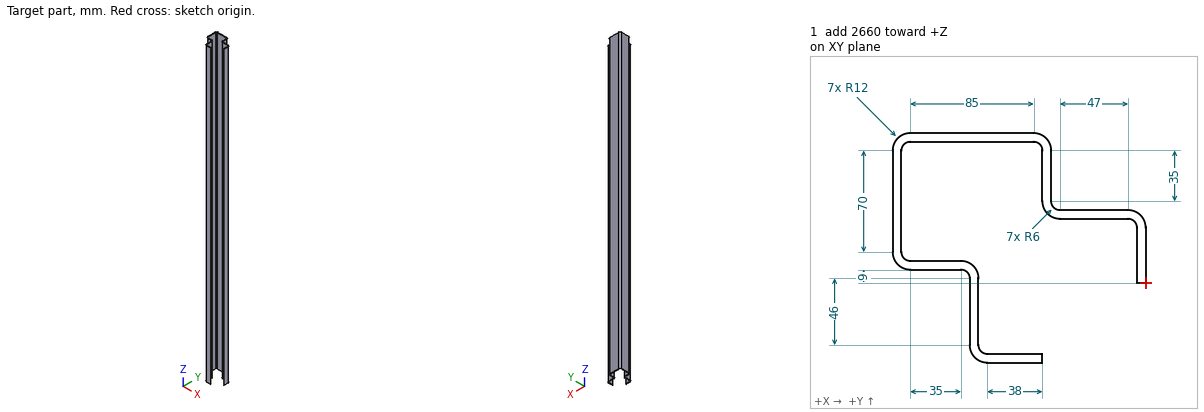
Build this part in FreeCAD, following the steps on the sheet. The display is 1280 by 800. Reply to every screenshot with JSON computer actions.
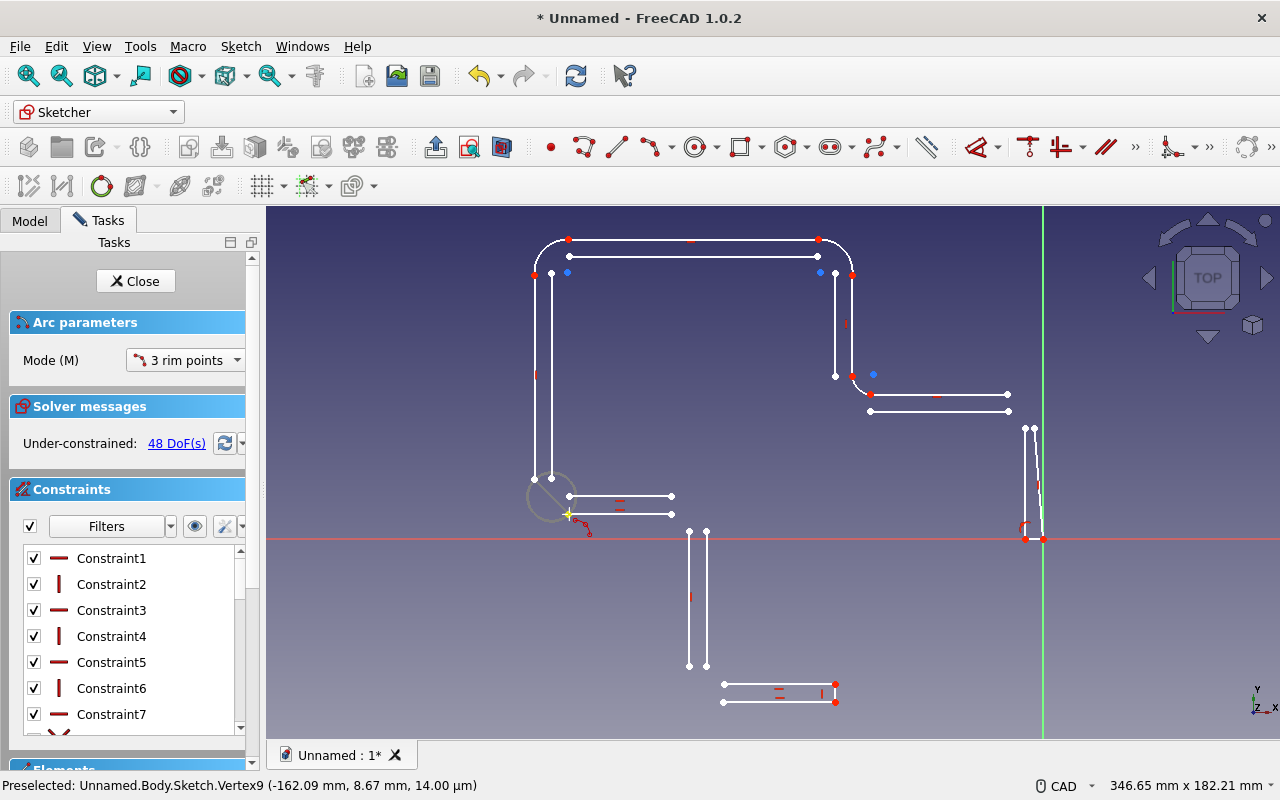
{"action": "scroll", "coordinate": [544, 503], "scroll_direction": "up", "scroll_amount": 3}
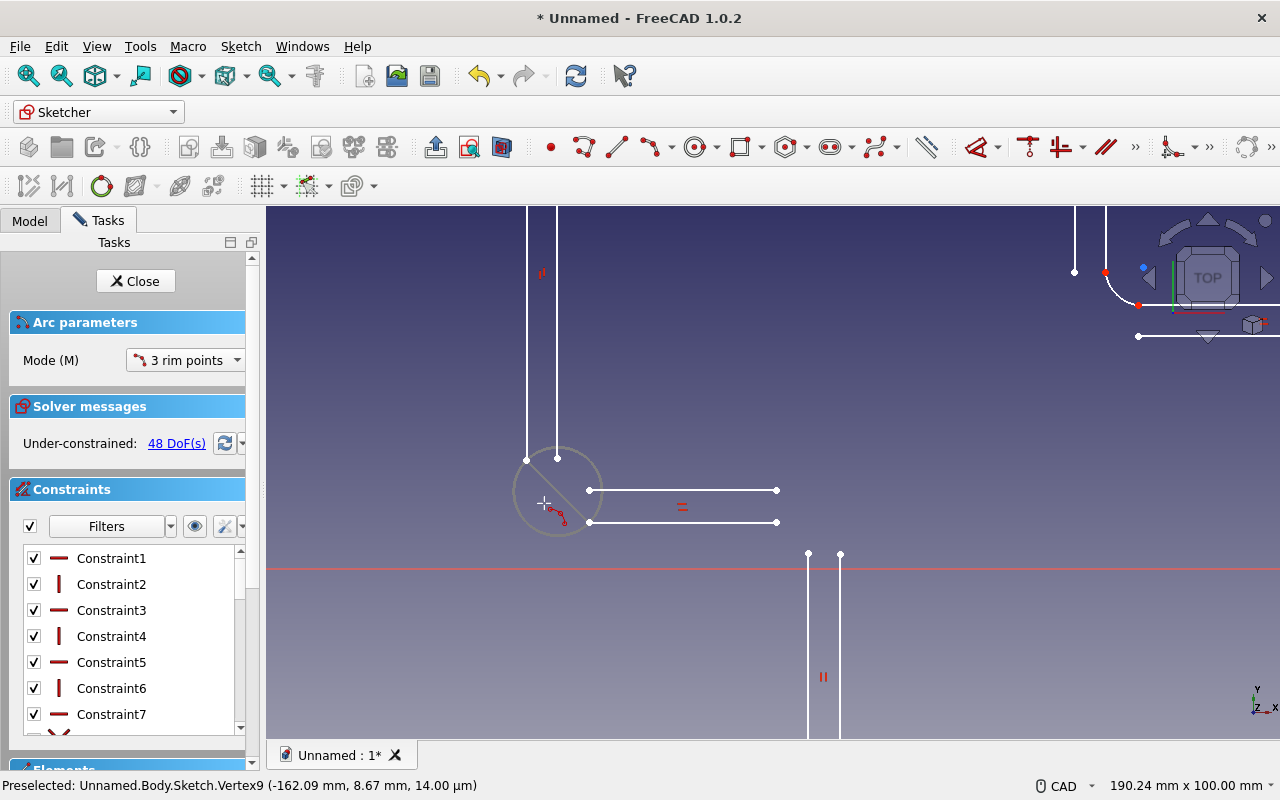
{"action": "left_click", "coordinate": [544, 502]}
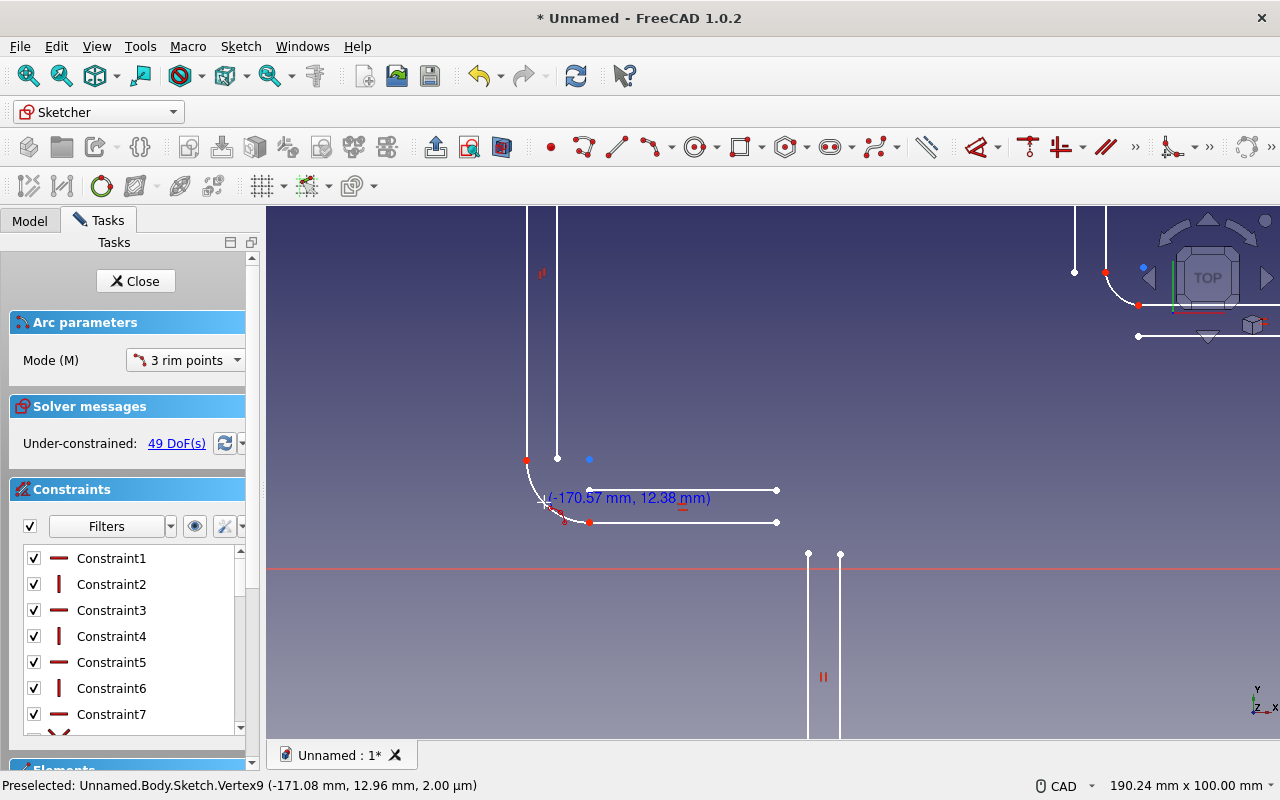
{"action": "left_click", "coordinate": [777, 523]}
{"action": "left_click", "coordinate": [808, 554]}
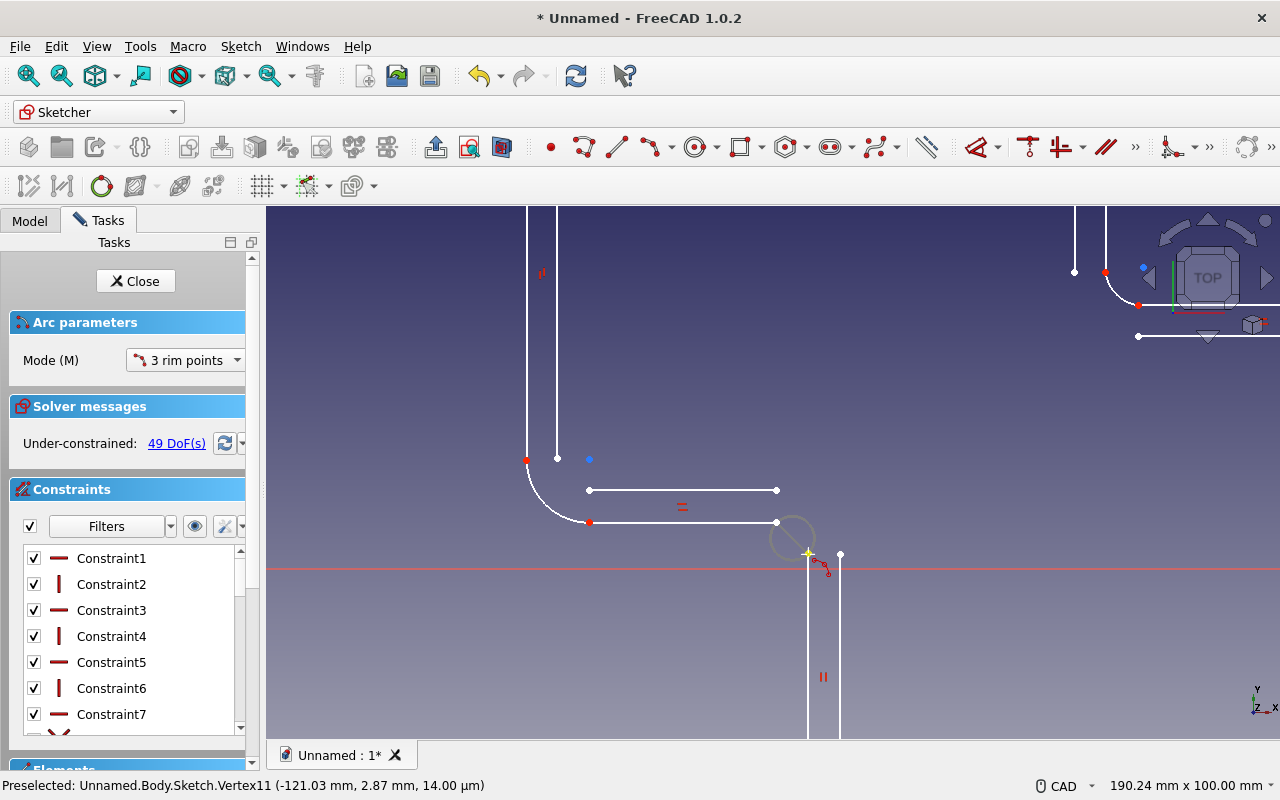
{"action": "scroll", "coordinate": [799, 530], "scroll_direction": "up", "scroll_amount": 3}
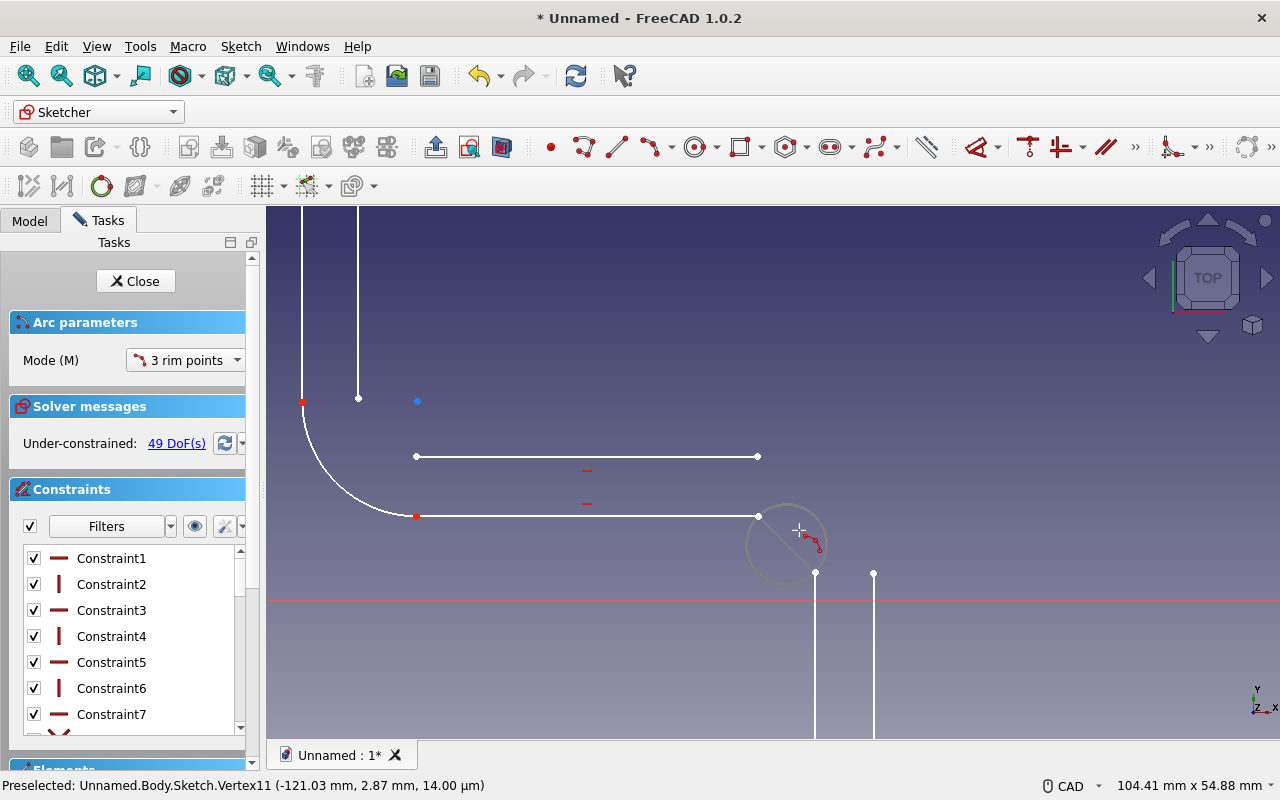
{"action": "left_click", "coordinate": [798, 530]}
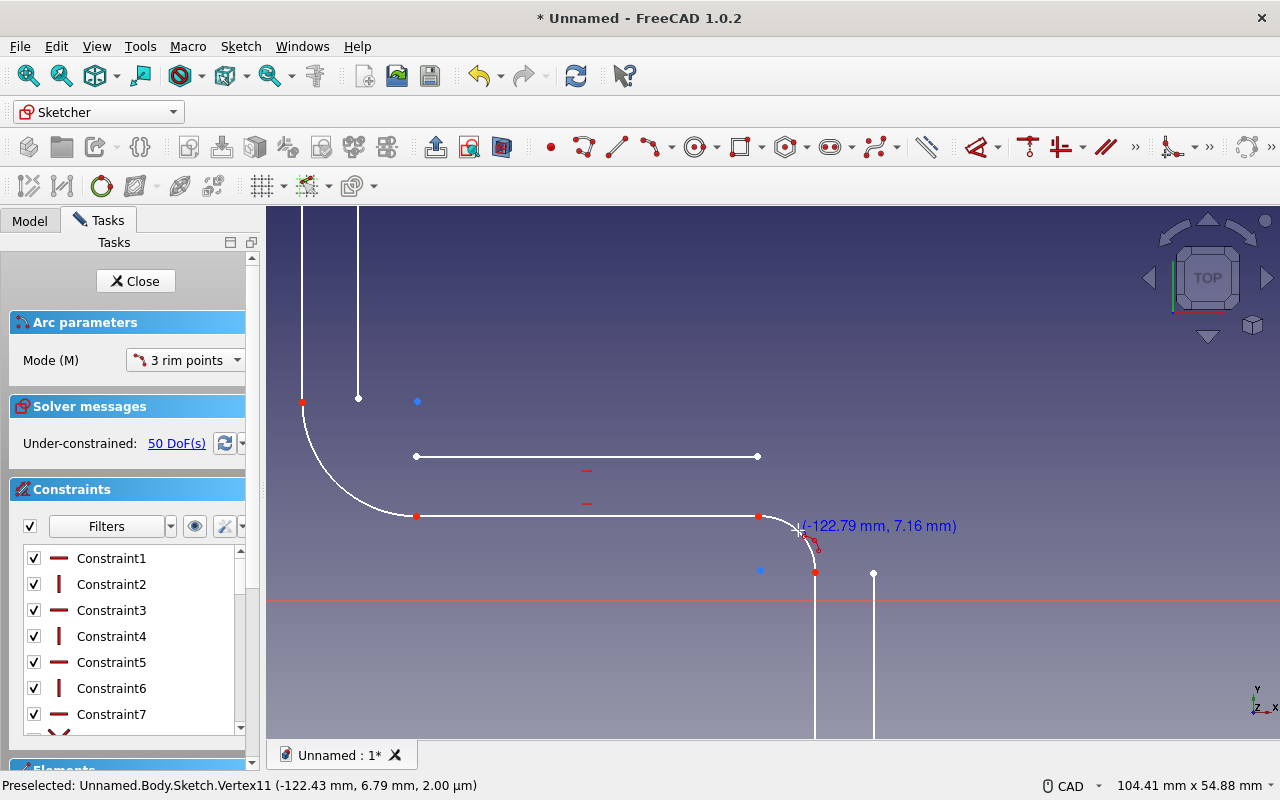
{"action": "scroll", "coordinate": [593, 499], "scroll_direction": "down", "scroll_amount": 8}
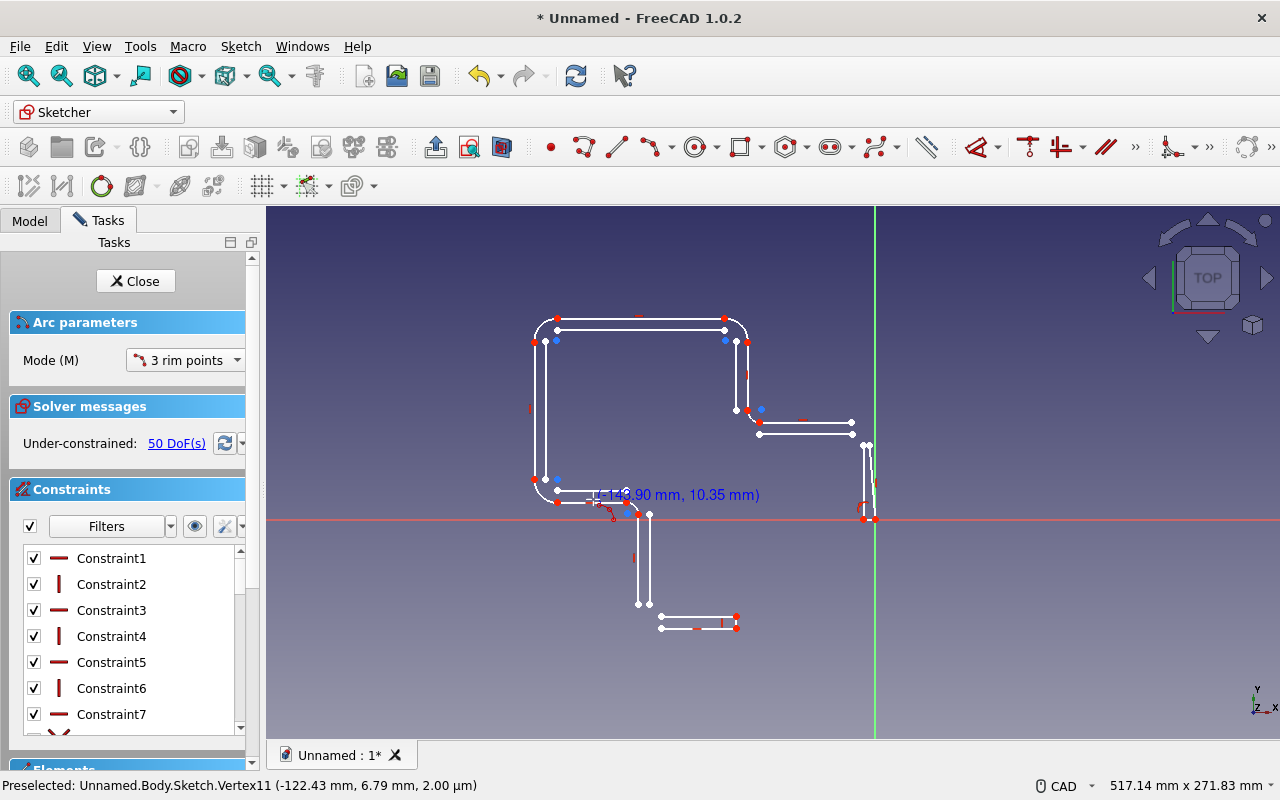
{"action": "scroll", "coordinate": [638, 604], "scroll_direction": "up", "scroll_amount": 2}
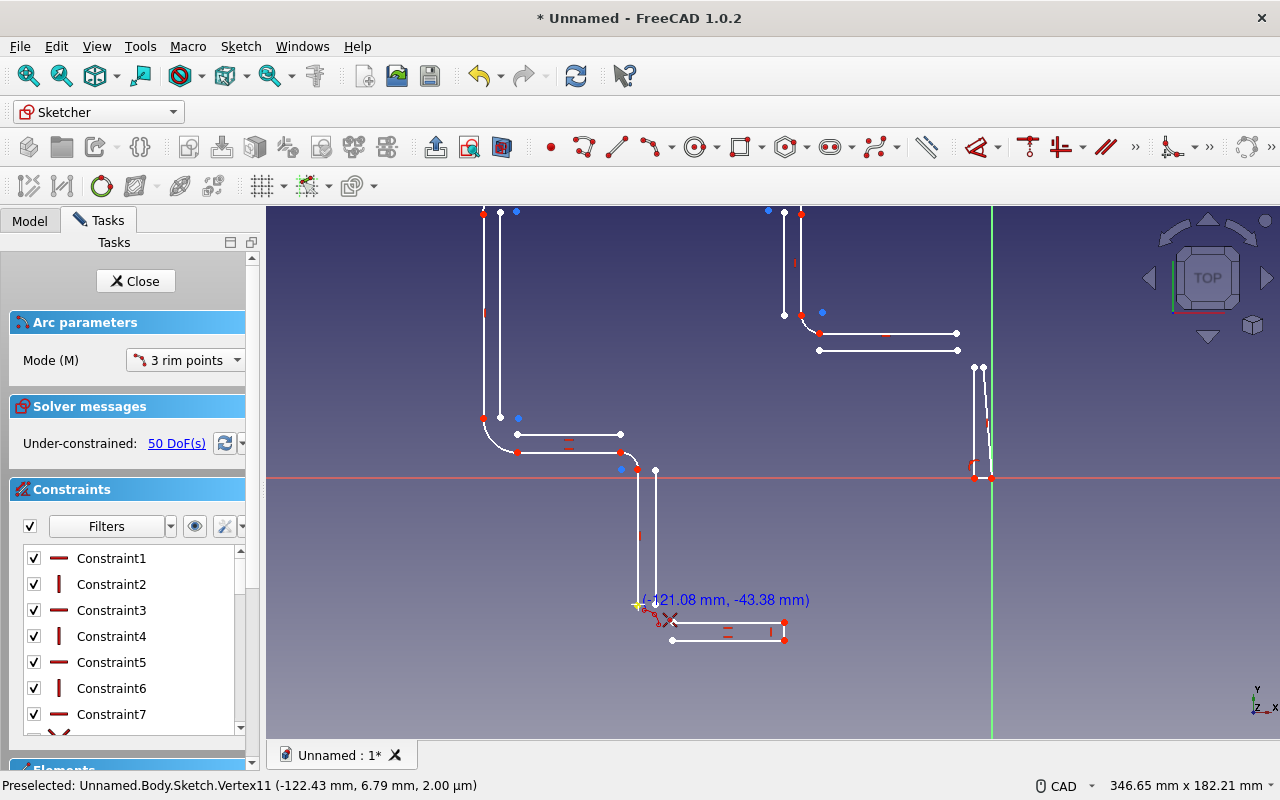
{"action": "left_click", "coordinate": [638, 605]}
{"action": "left_click", "coordinate": [672, 641]}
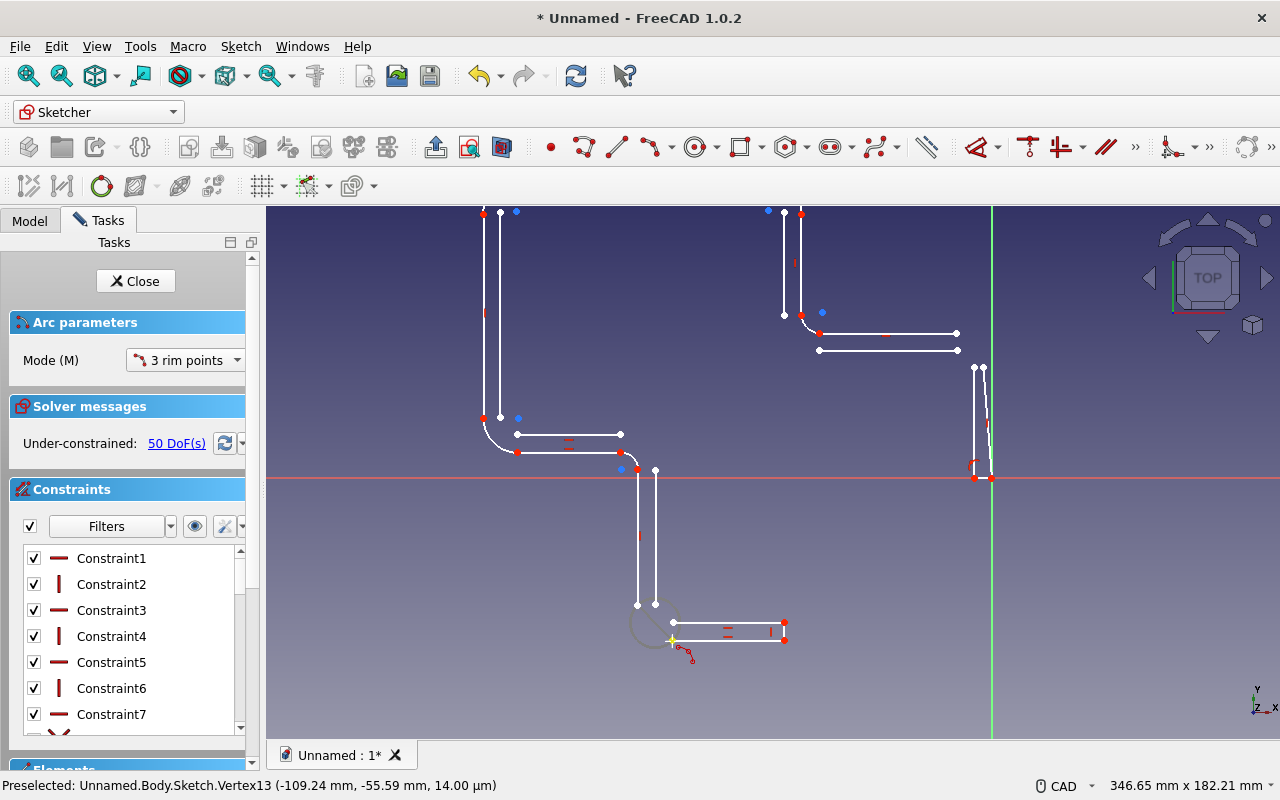
{"action": "scroll", "coordinate": [648, 629], "scroll_direction": "up", "scroll_amount": 3}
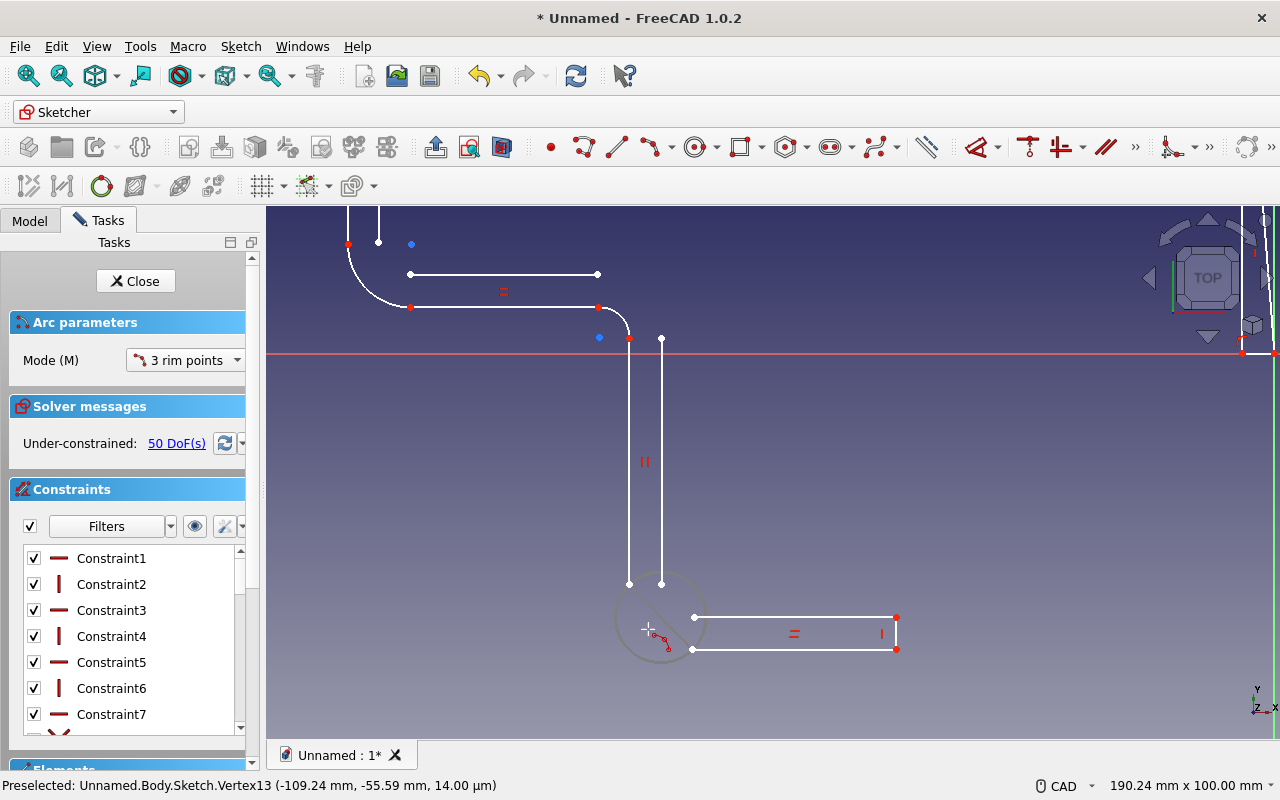
{"action": "left_click", "coordinate": [648, 628]}